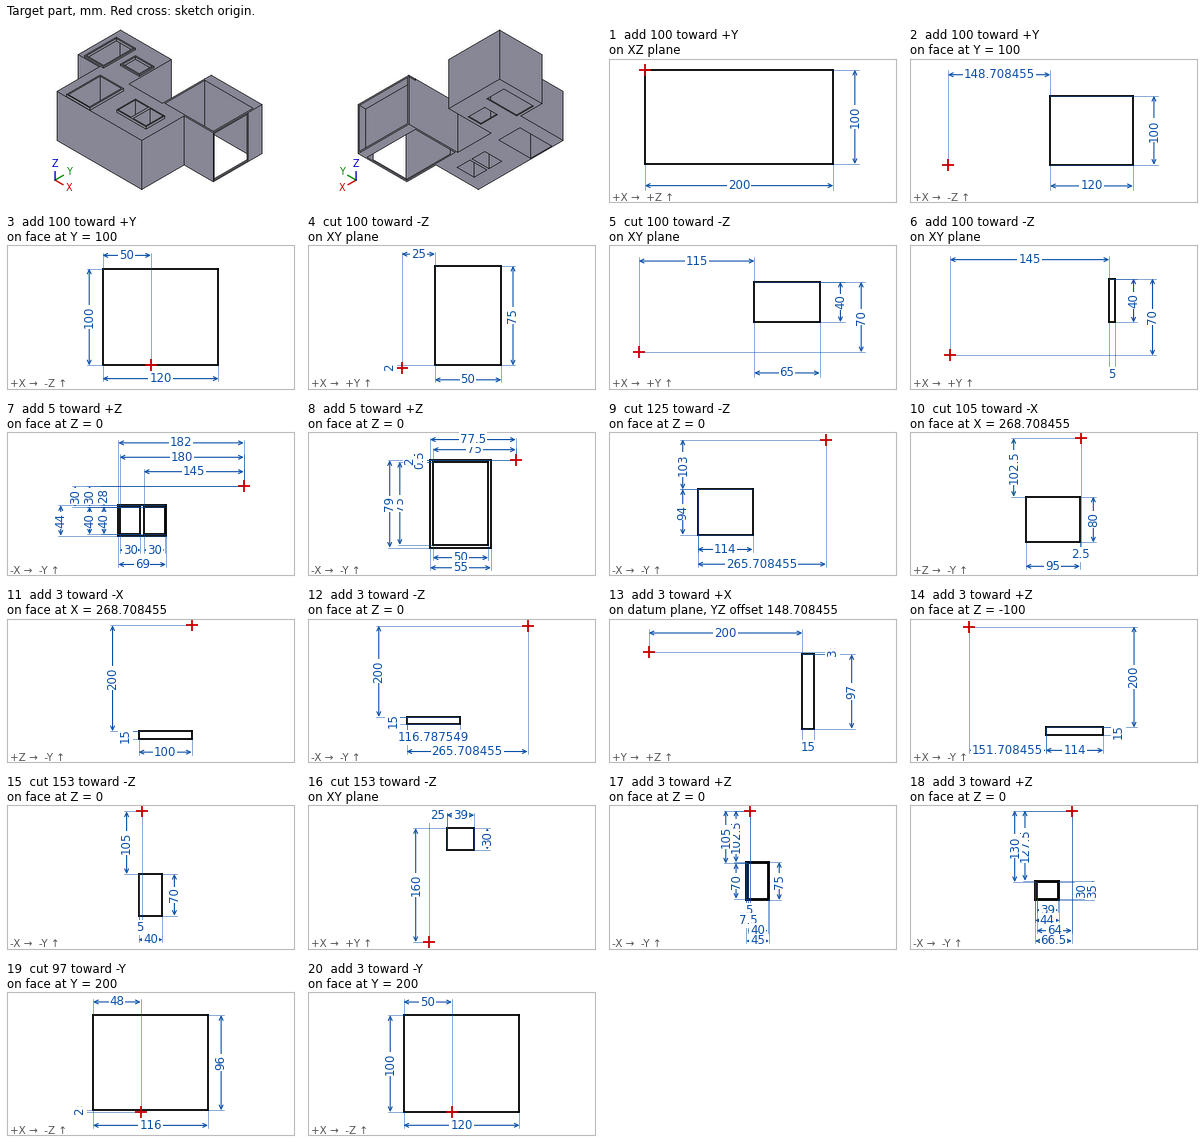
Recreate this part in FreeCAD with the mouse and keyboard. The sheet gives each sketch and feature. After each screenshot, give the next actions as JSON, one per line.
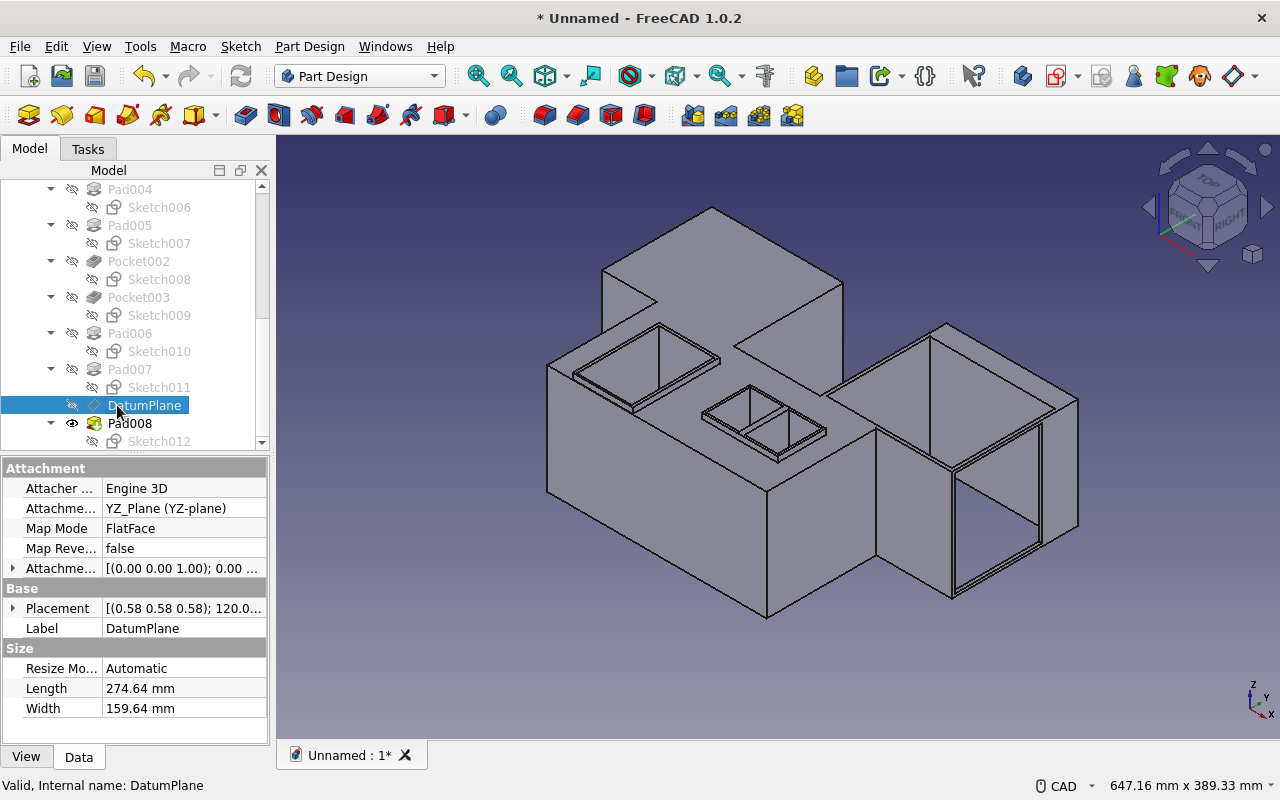
{"action": "key", "text": "5"}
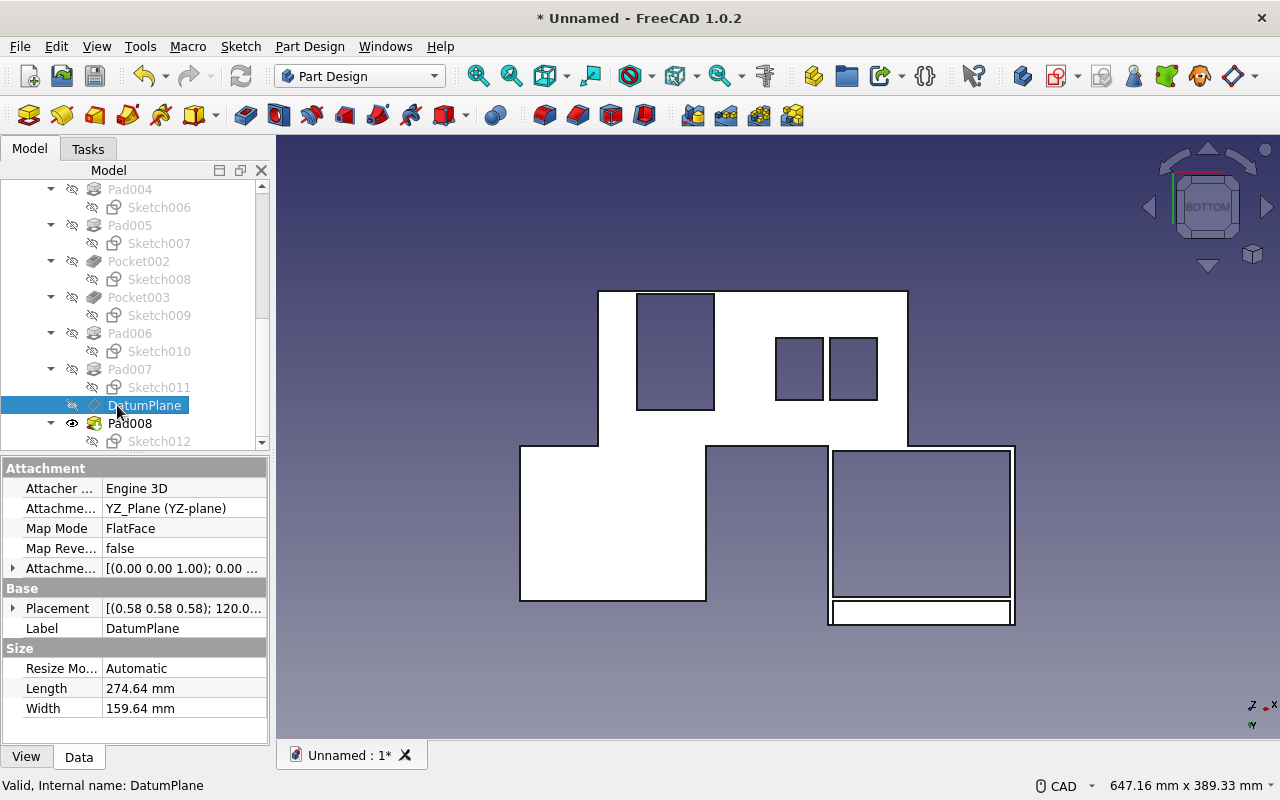
{"action": "left_click", "coordinate": [626, 504]}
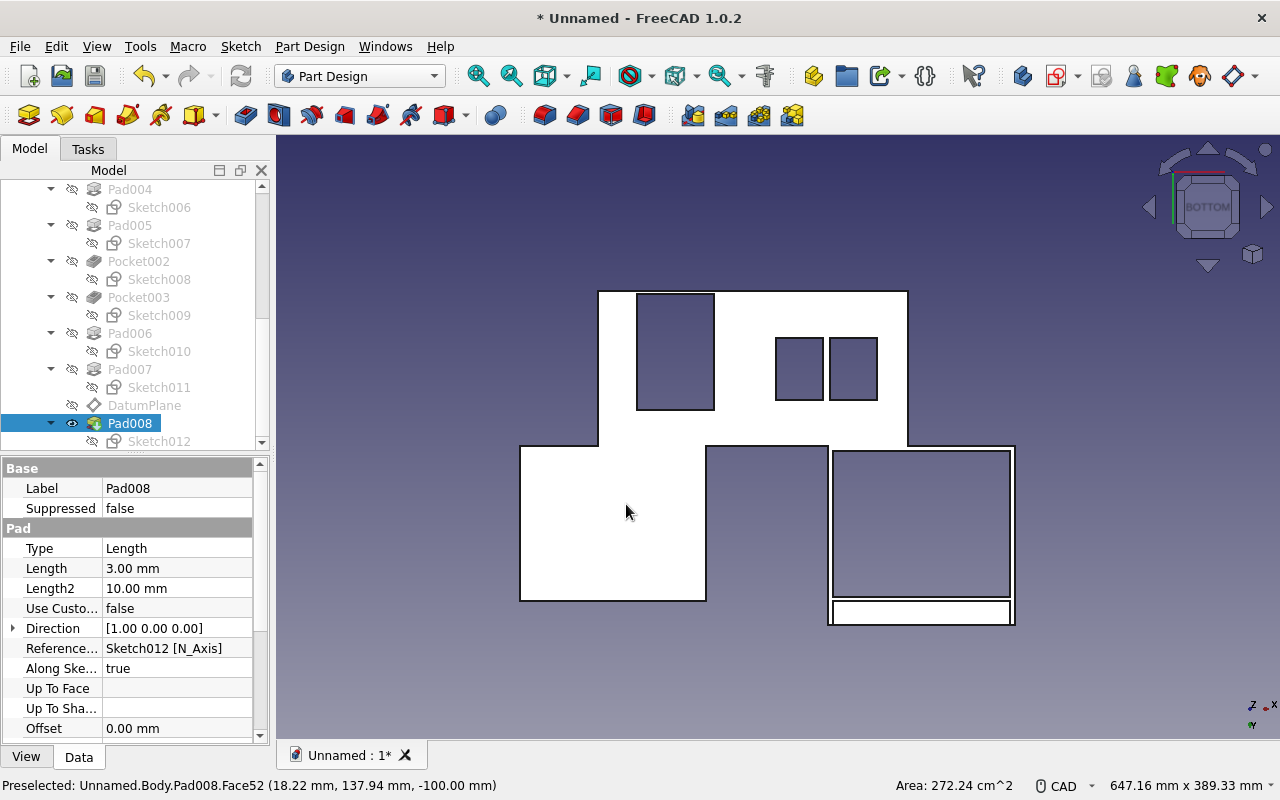
{"action": "left_click", "coordinate": [1056, 76]}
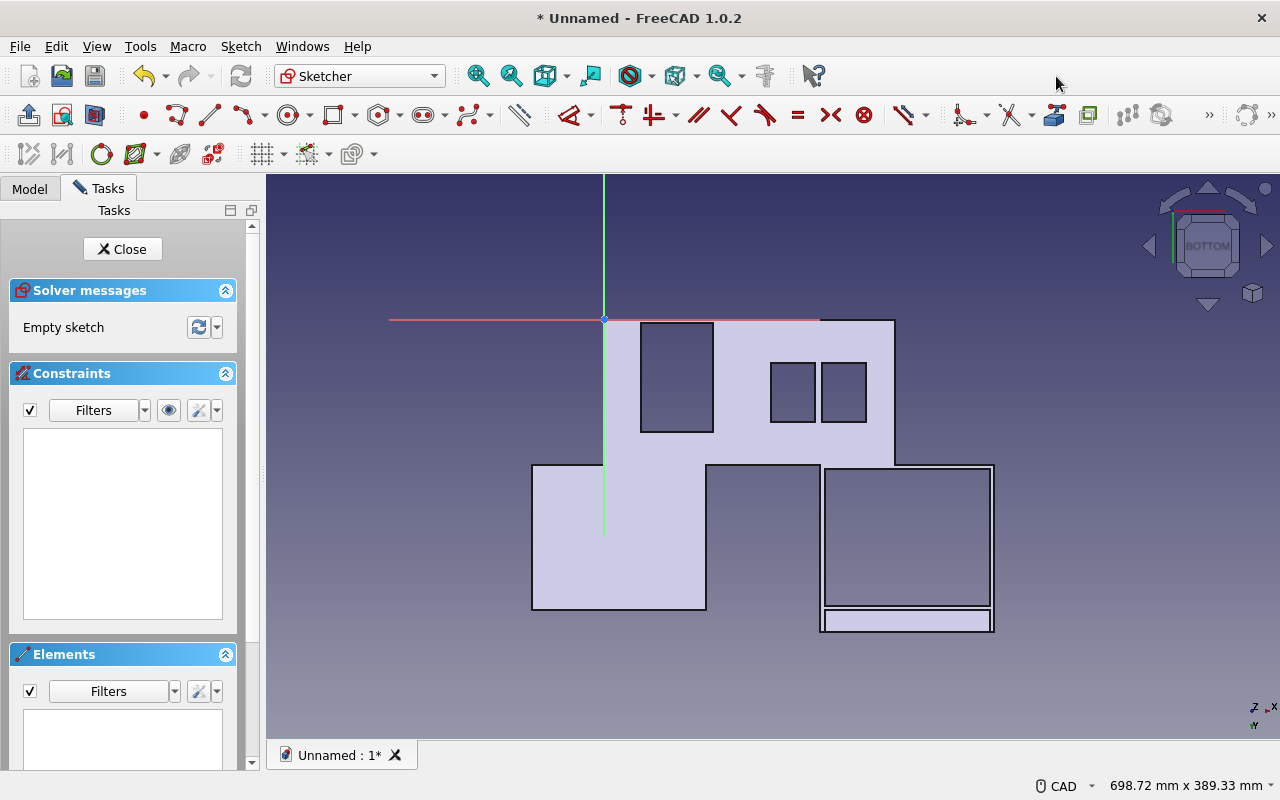
{"action": "left_click", "coordinate": [332, 116]}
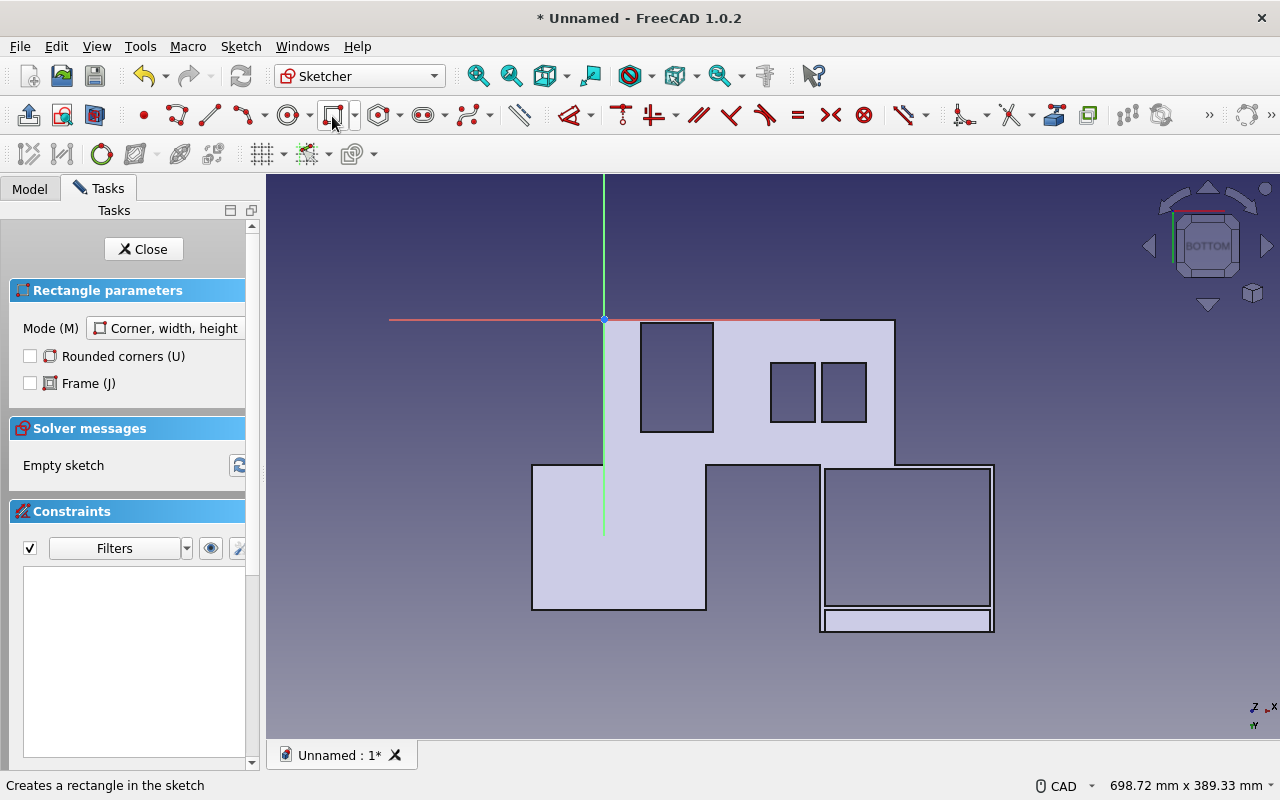
{"action": "left_click", "coordinate": [825, 610]}
{"action": "mouse_move", "coordinate": [990, 632]}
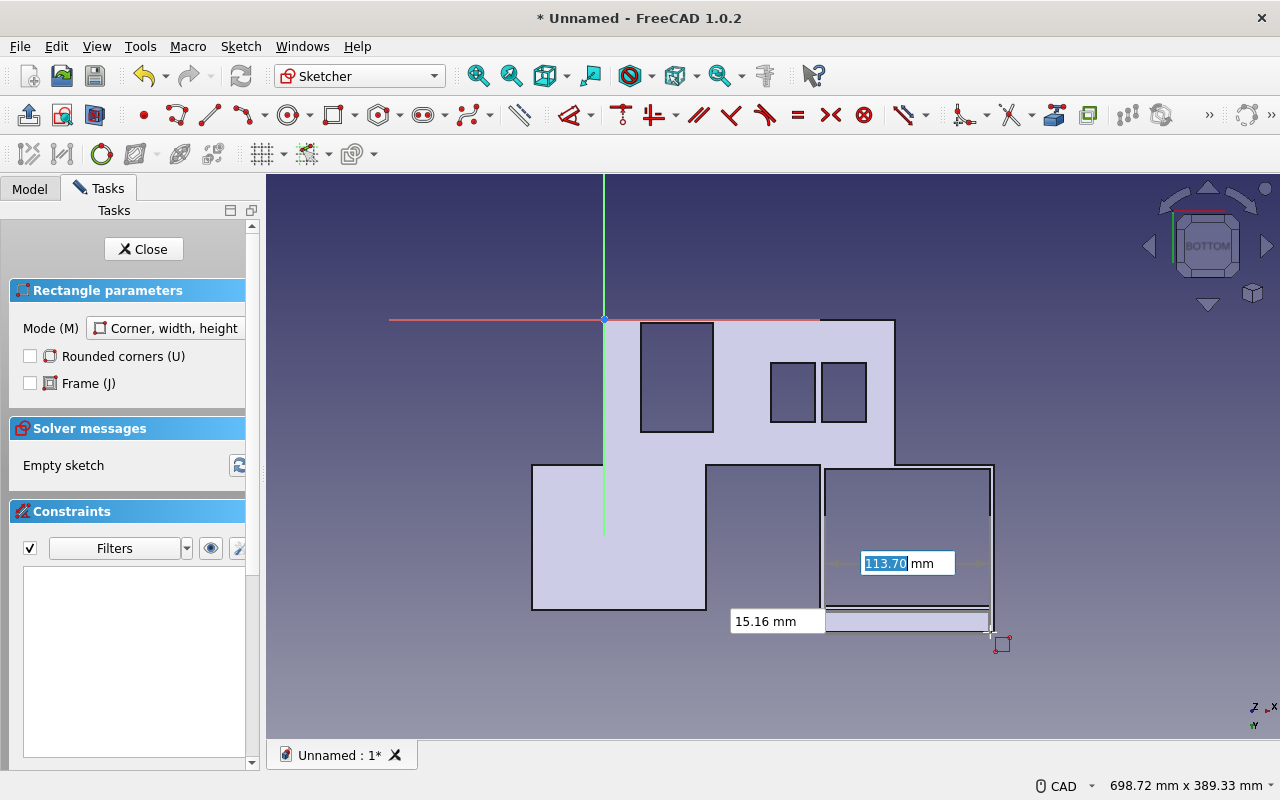
{"action": "type", "text": "114"}
{"action": "key", "text": "Tab"}
{"action": "type", "text": "15"}
{"action": "key", "text": "Return"}
{"action": "key", "text": "Escape"}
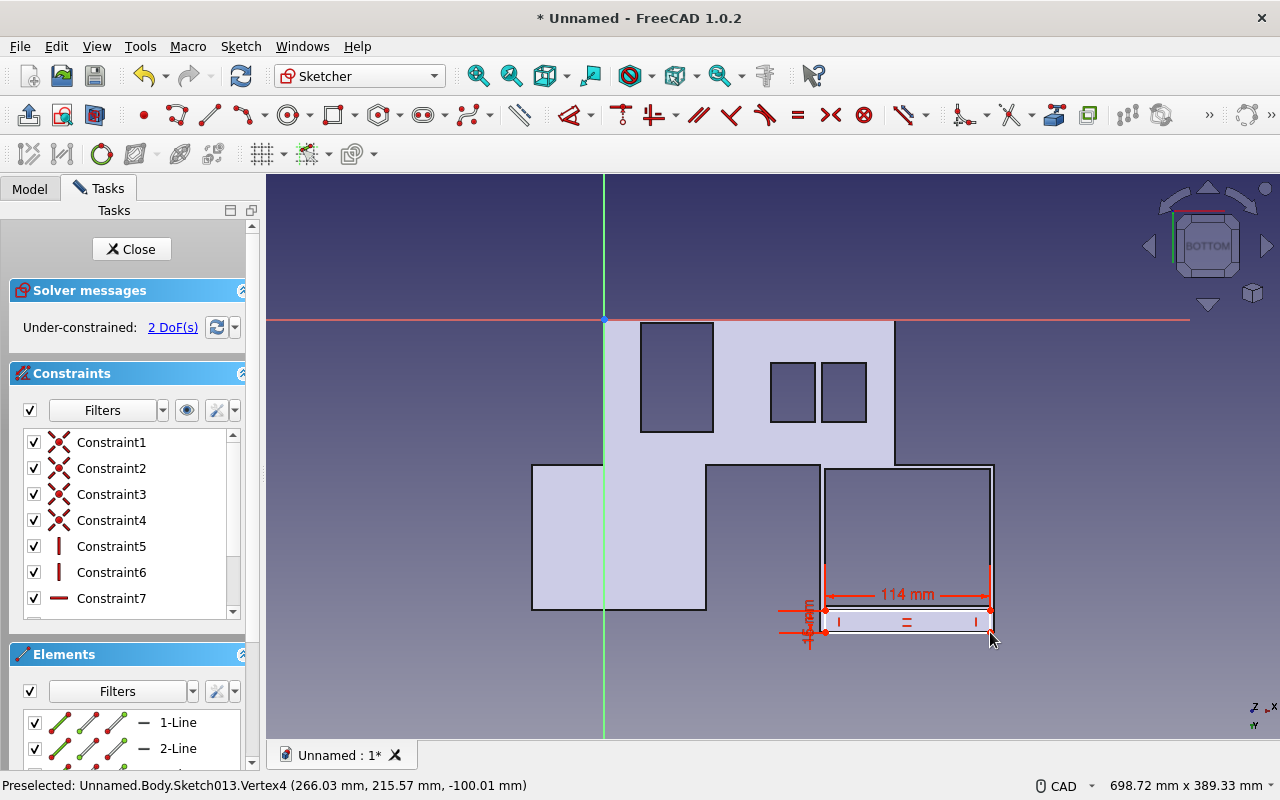
{"action": "left_click", "coordinate": [568, 116]}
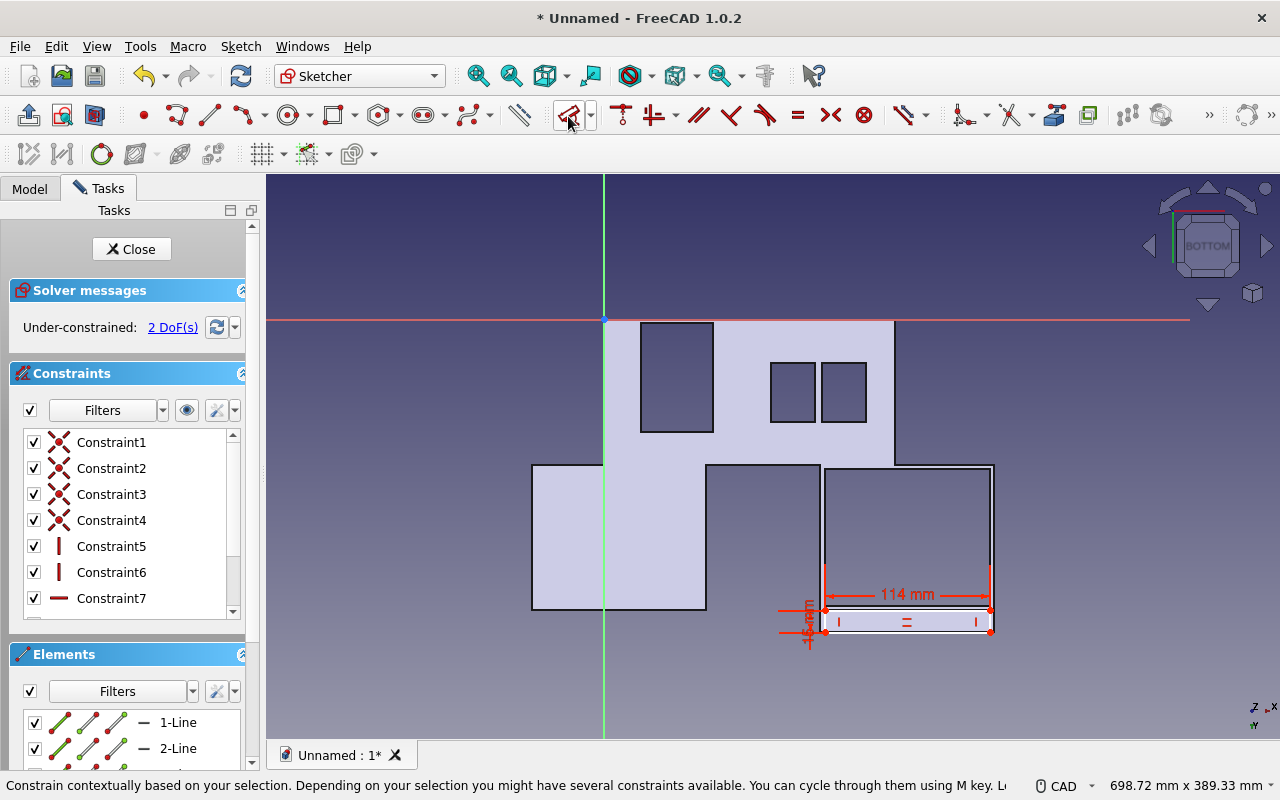
{"action": "left_click", "coordinate": [825, 611]}
{"action": "left_click", "coordinate": [570, 465]}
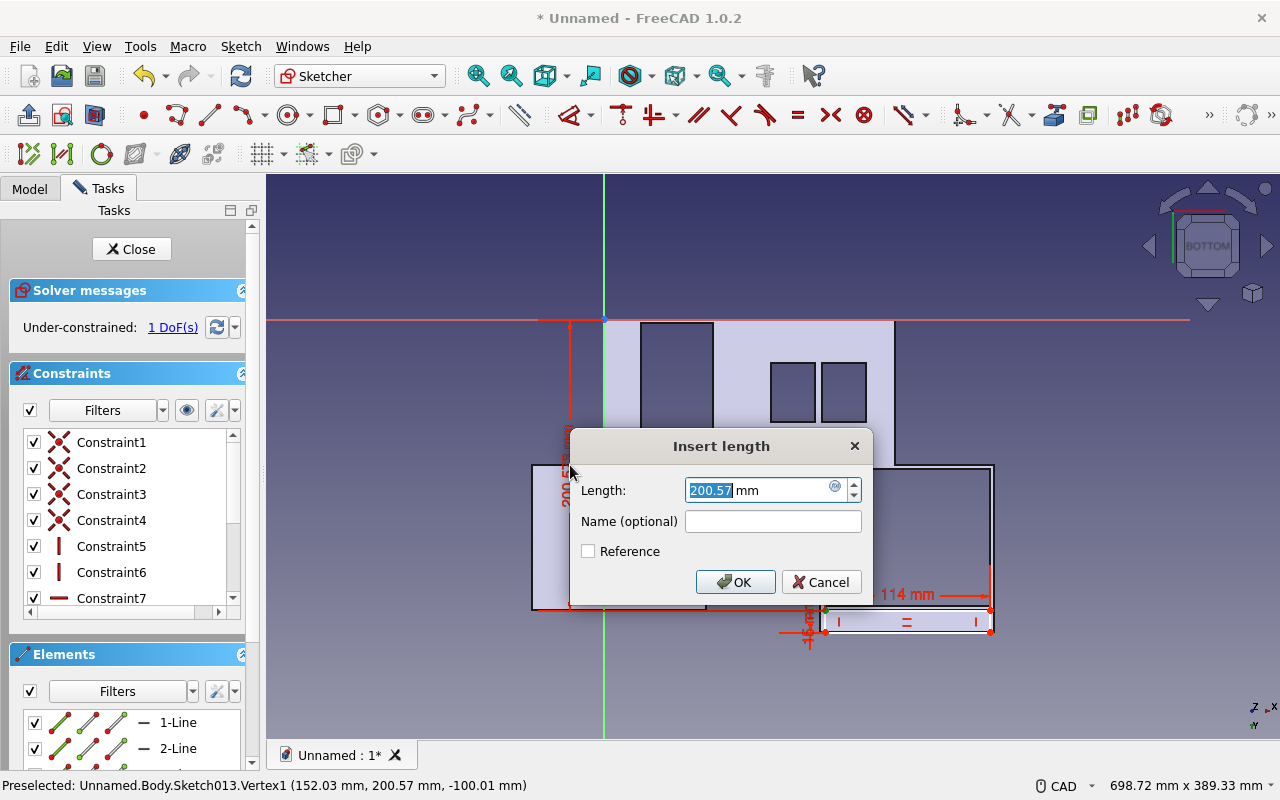
{"action": "type", "text": "200"}
{"action": "key", "text": "Return"}